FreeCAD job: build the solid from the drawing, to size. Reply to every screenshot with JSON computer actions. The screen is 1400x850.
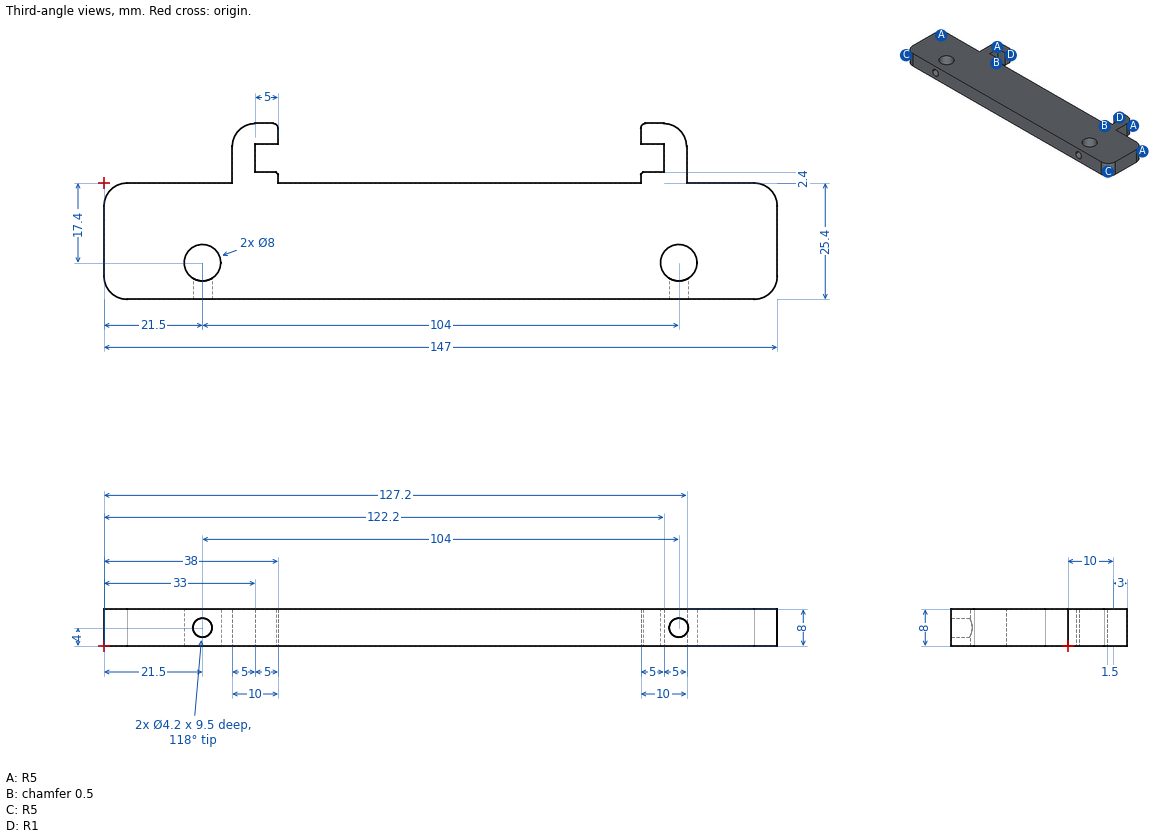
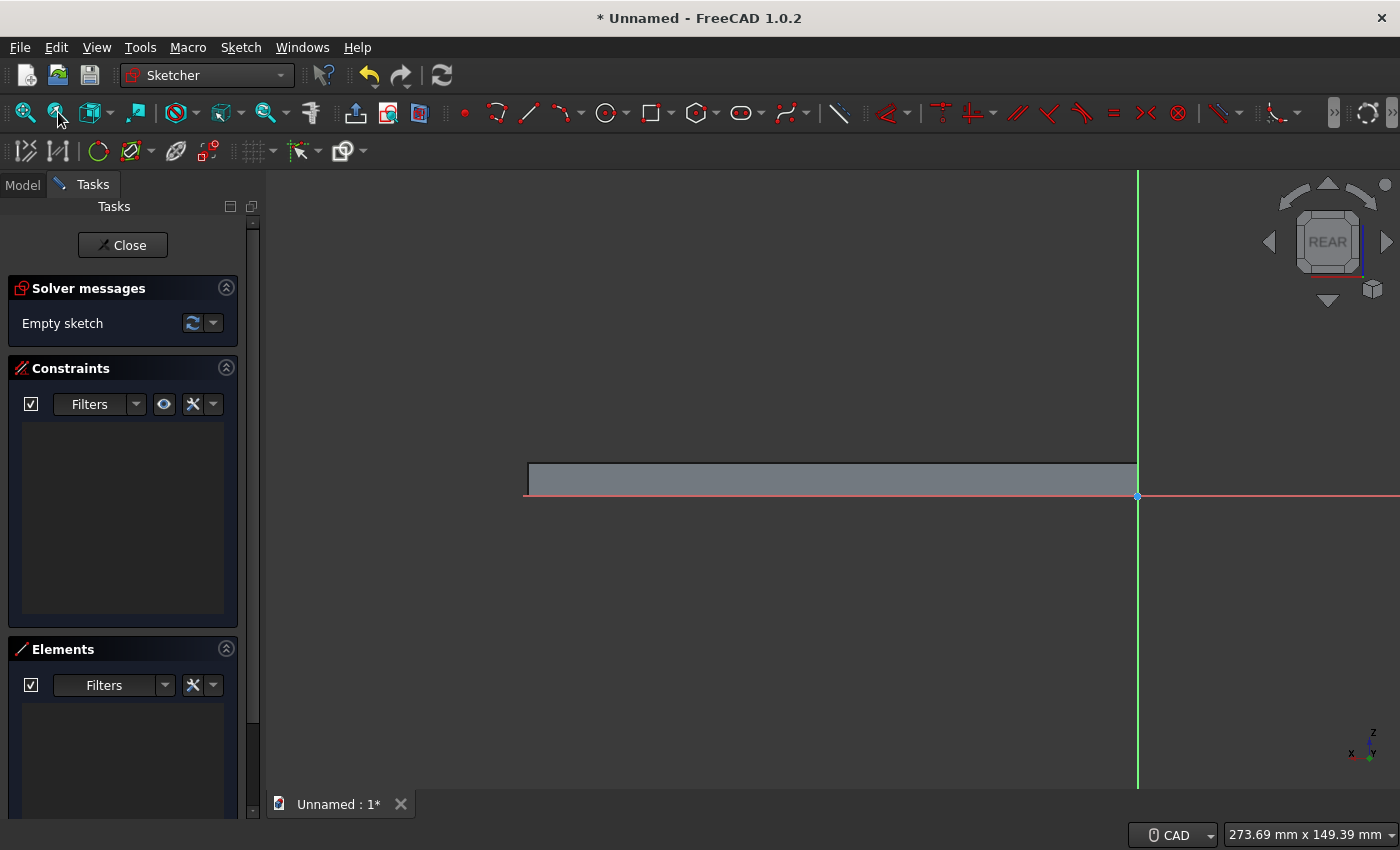
{"action": "left_click", "coordinate": [652, 114]}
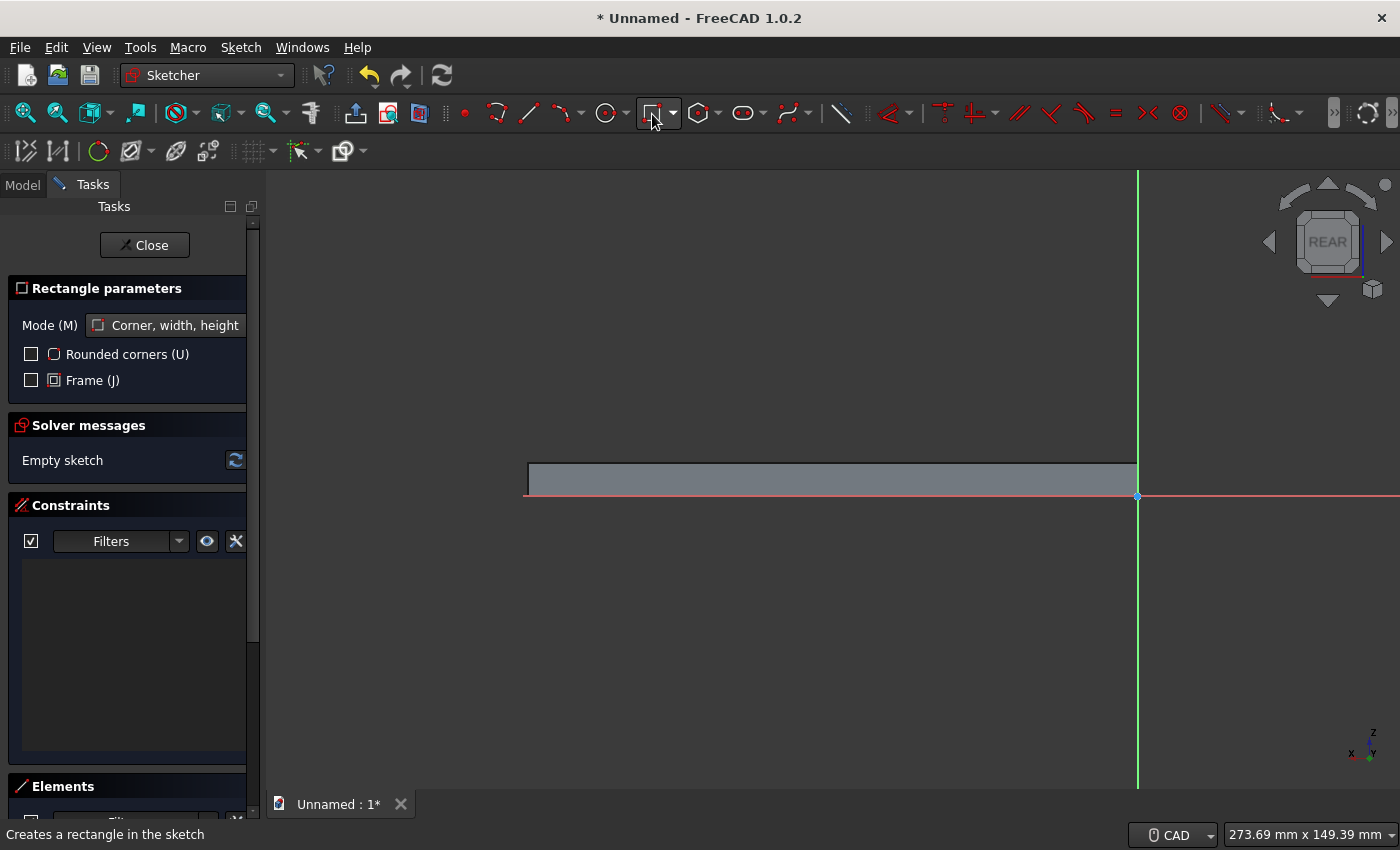
{"action": "left_click", "coordinate": [610, 463]}
{"action": "left_click", "coordinate": [631, 496]}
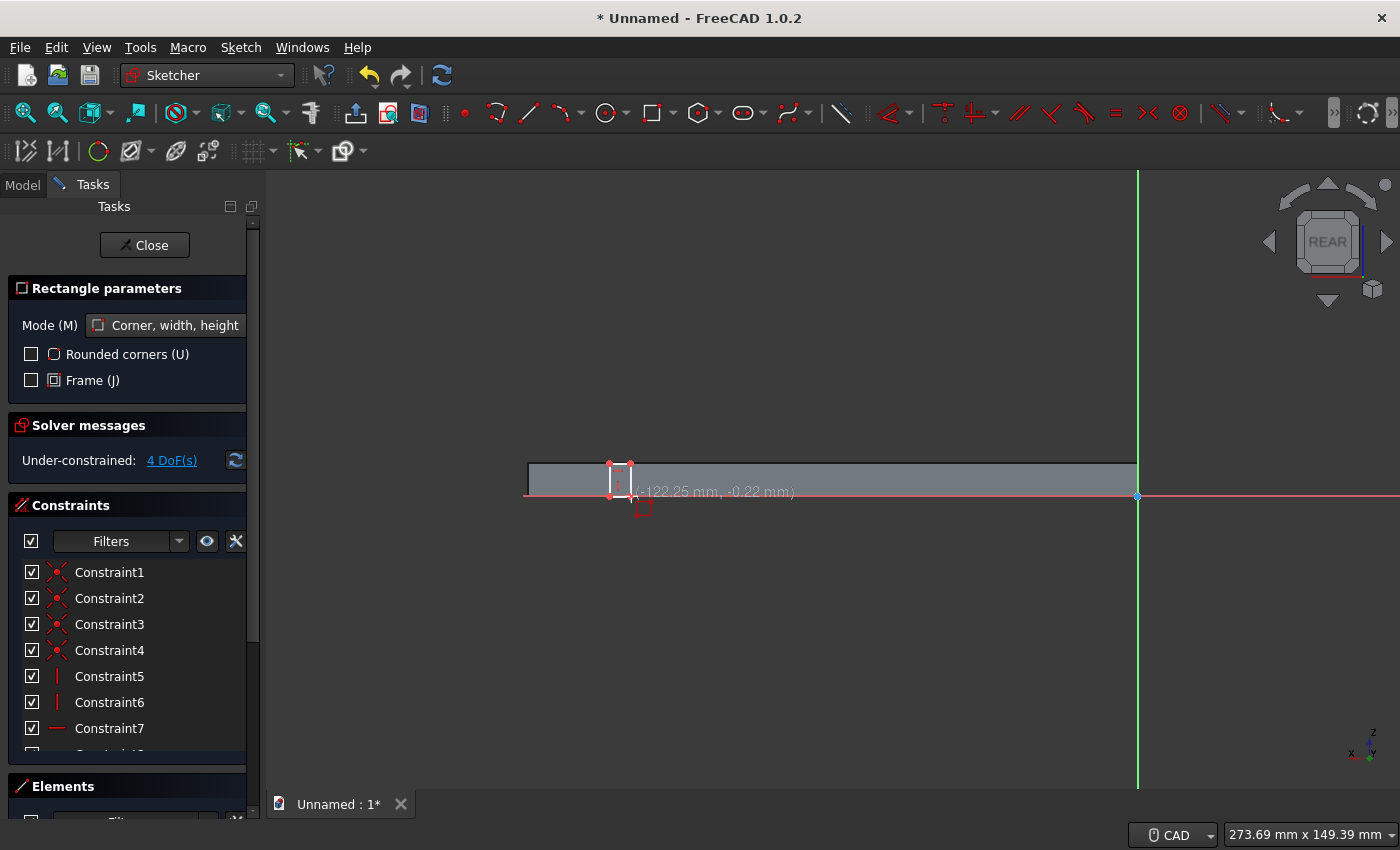
{"action": "left_click", "coordinate": [1001, 463]}
{"action": "left_click", "coordinate": [1022, 496]}
{"action": "key", "text": "Escape"}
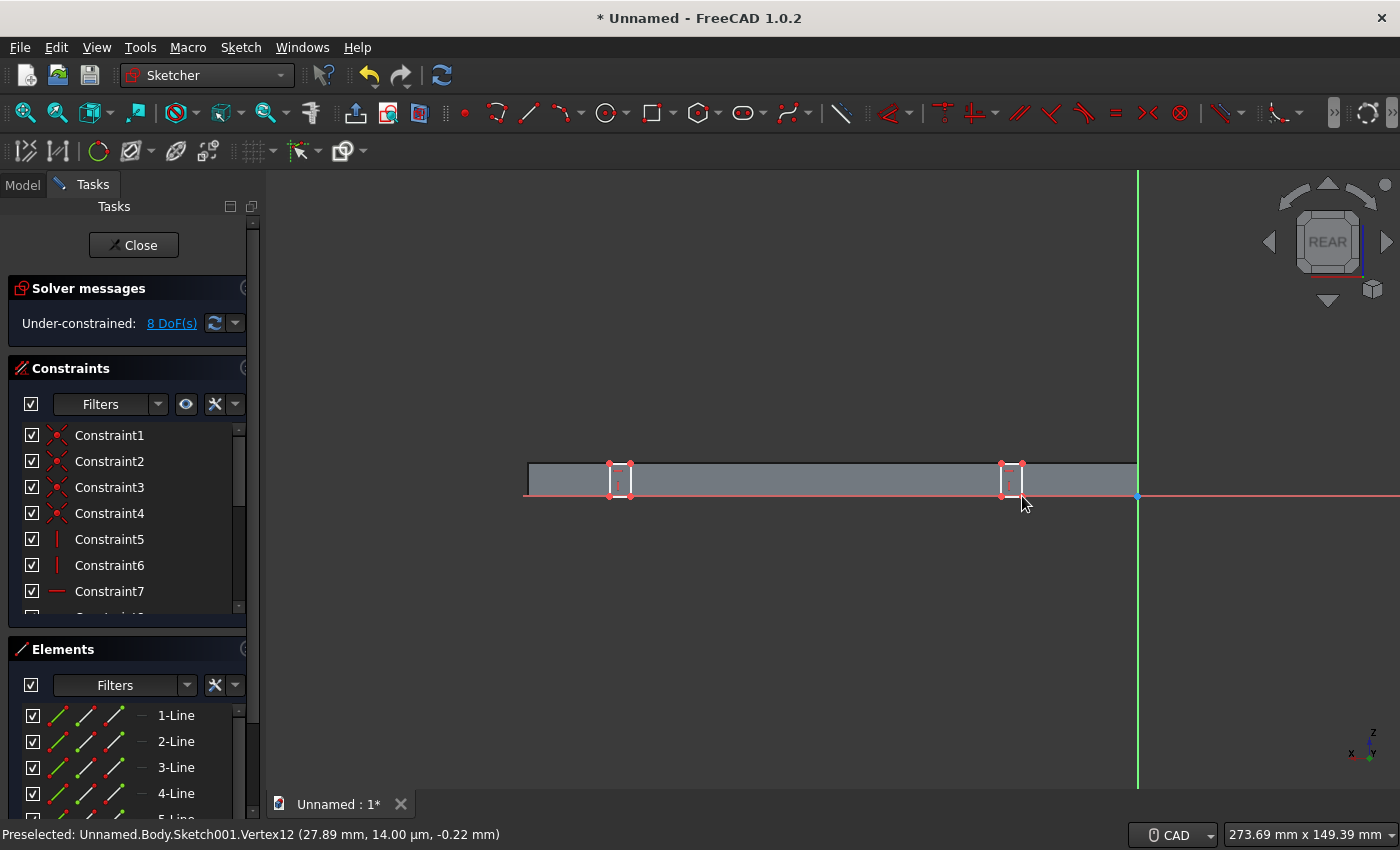
{"action": "left_click", "coordinate": [610, 497]}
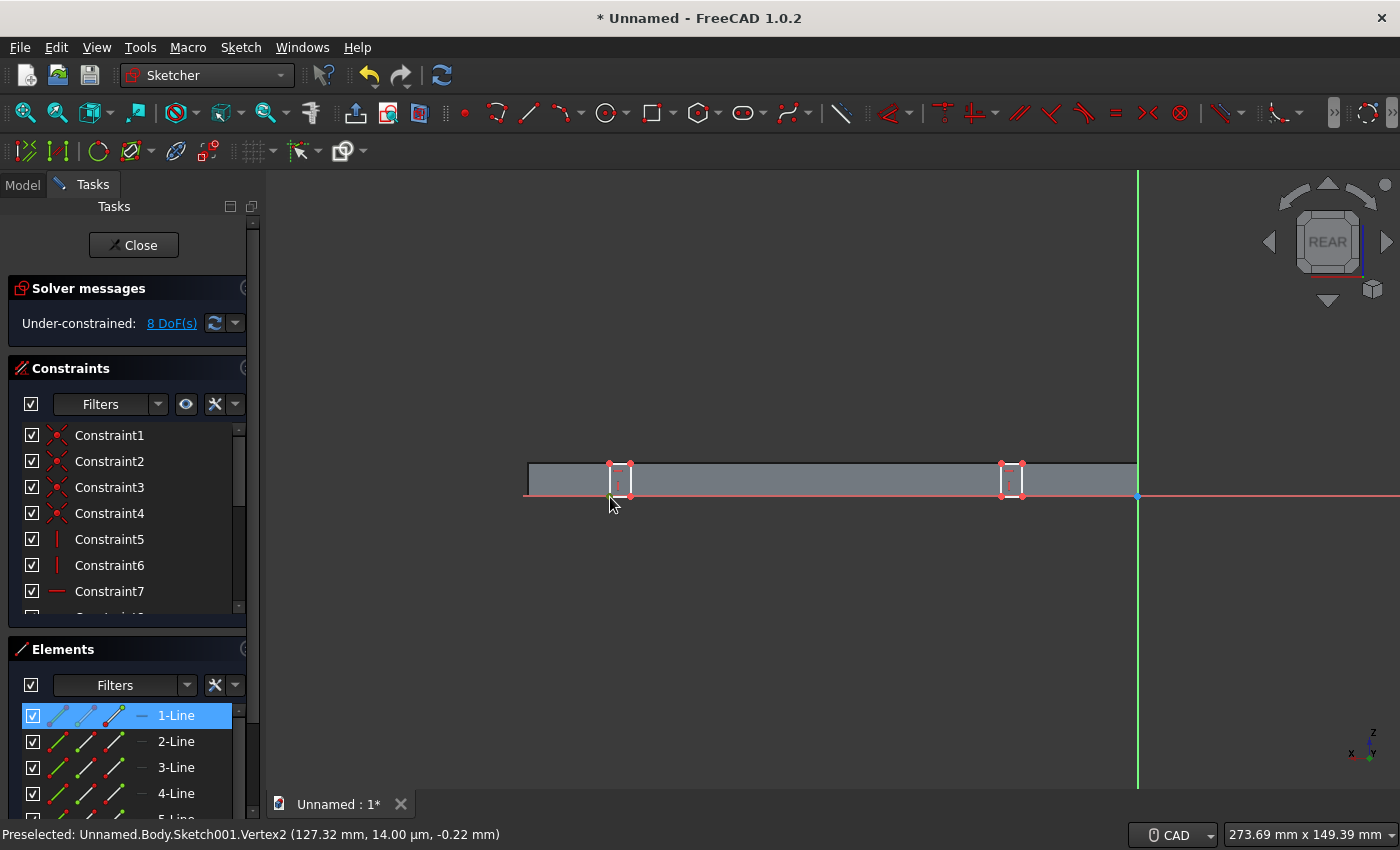
{"action": "left_click", "coordinate": [563, 496]}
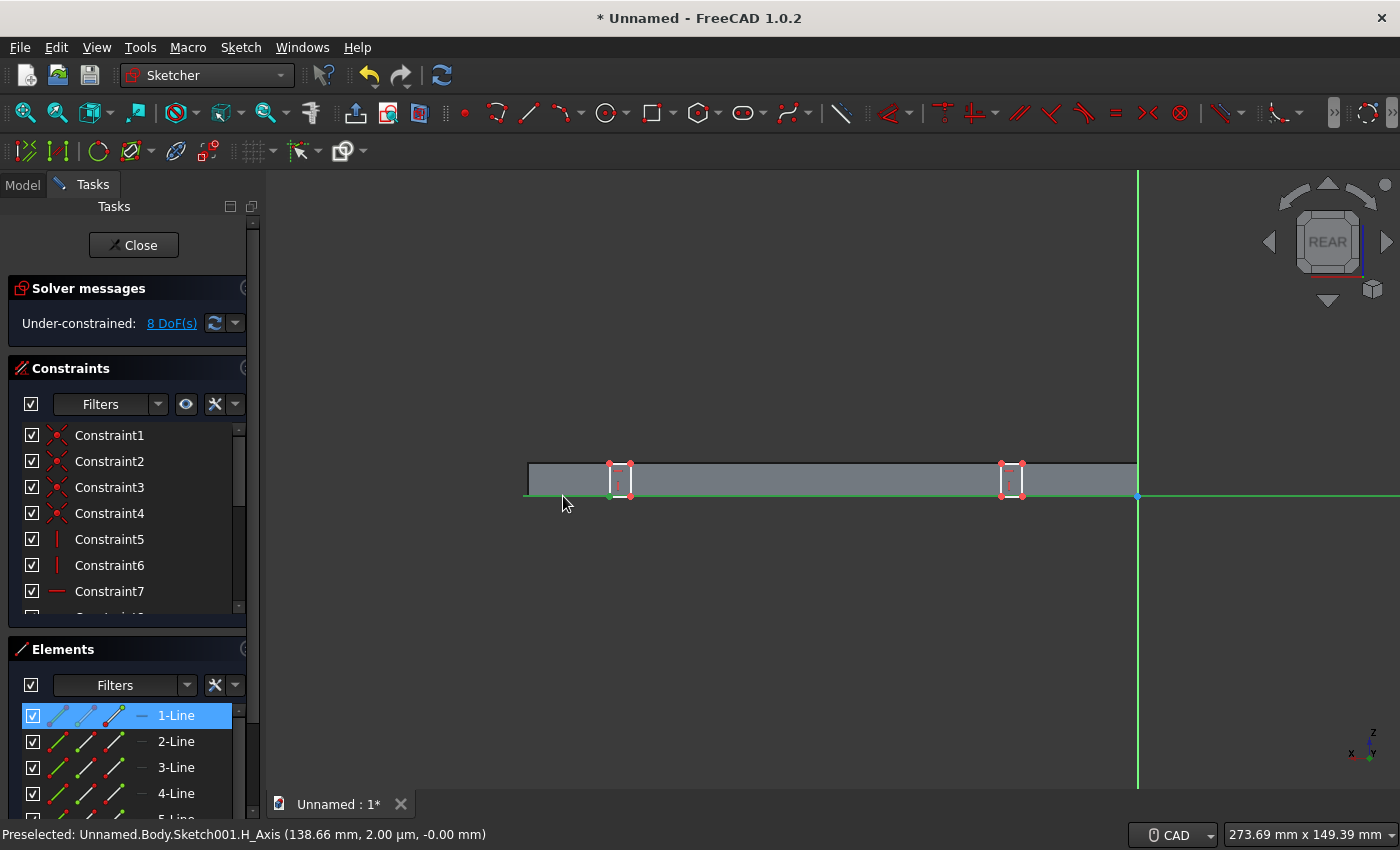
{"action": "key", "text": "c"}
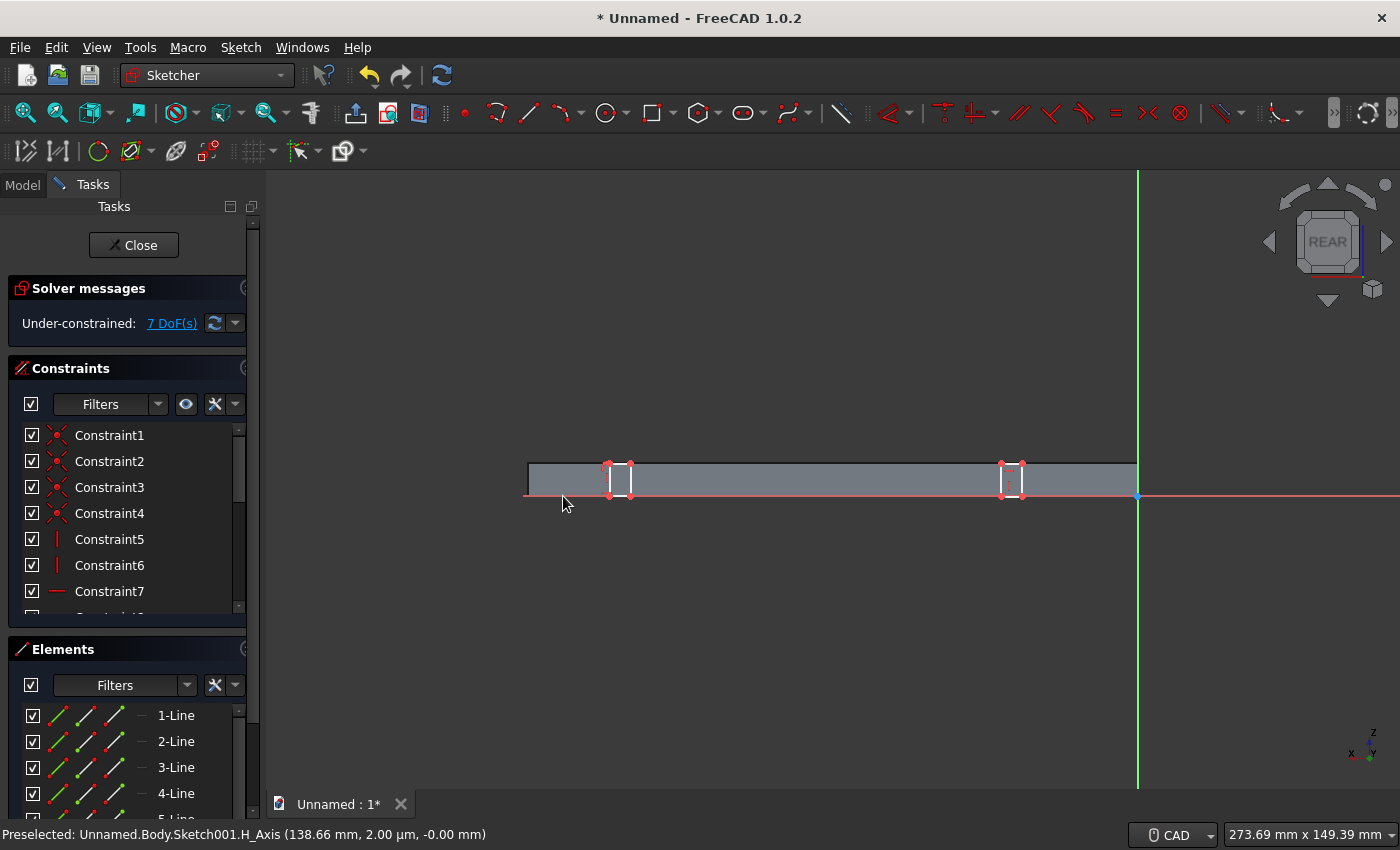
{"action": "left_click", "coordinate": [1001, 497]}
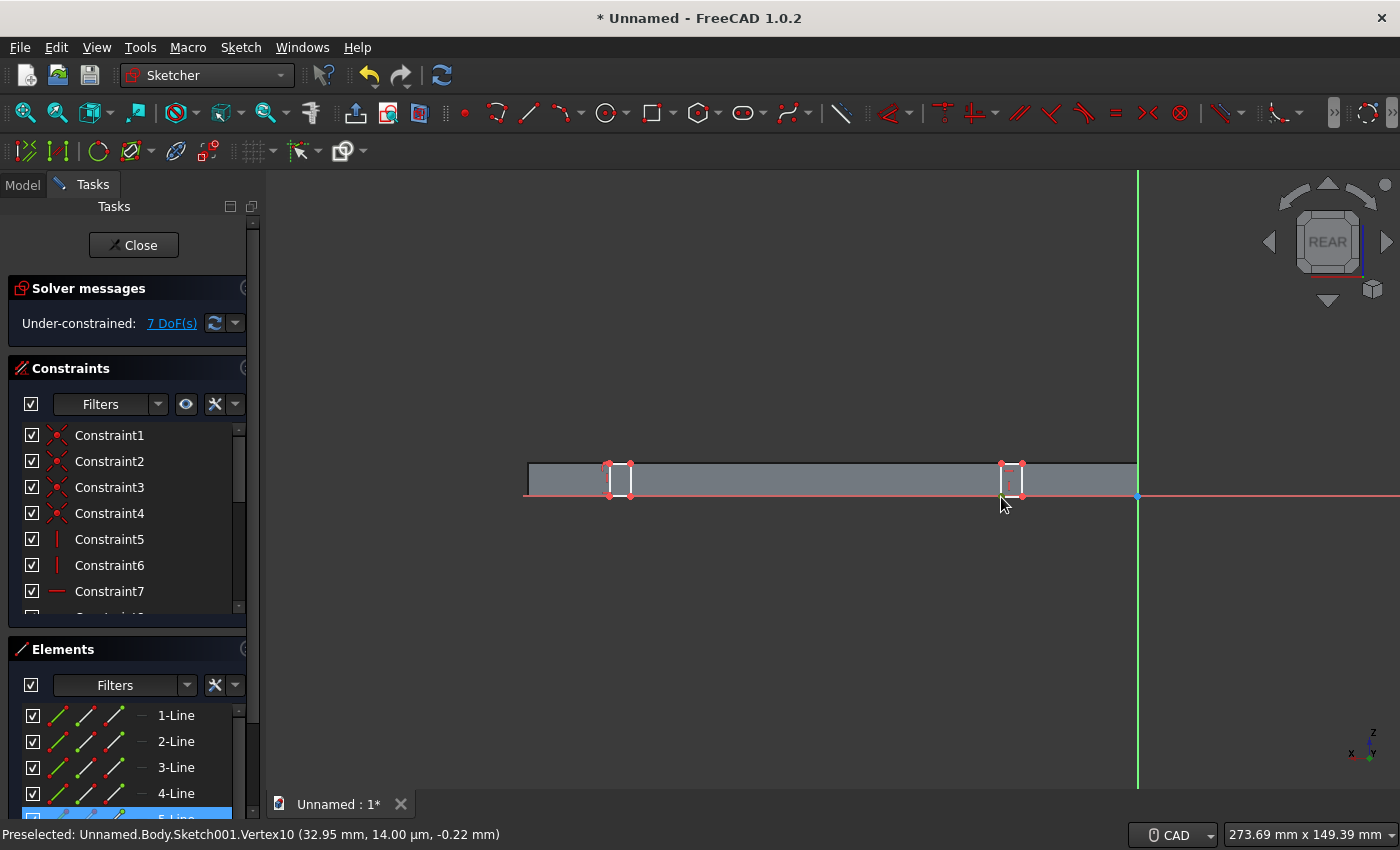
{"action": "left_click", "coordinate": [563, 496]}